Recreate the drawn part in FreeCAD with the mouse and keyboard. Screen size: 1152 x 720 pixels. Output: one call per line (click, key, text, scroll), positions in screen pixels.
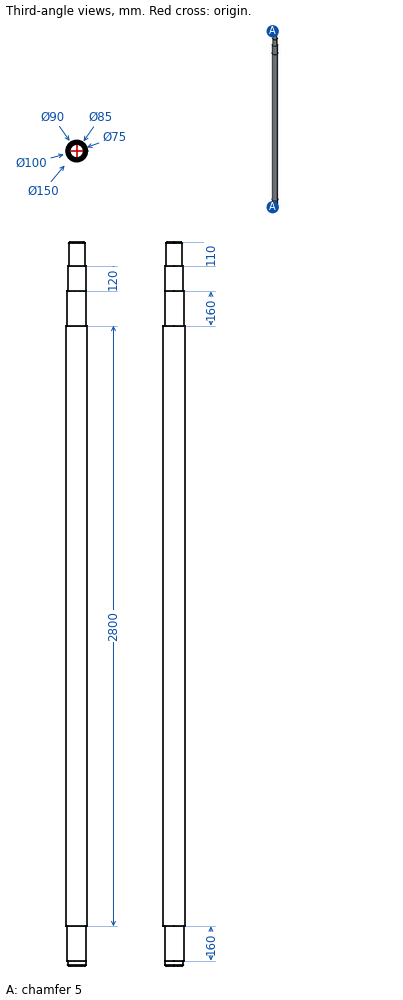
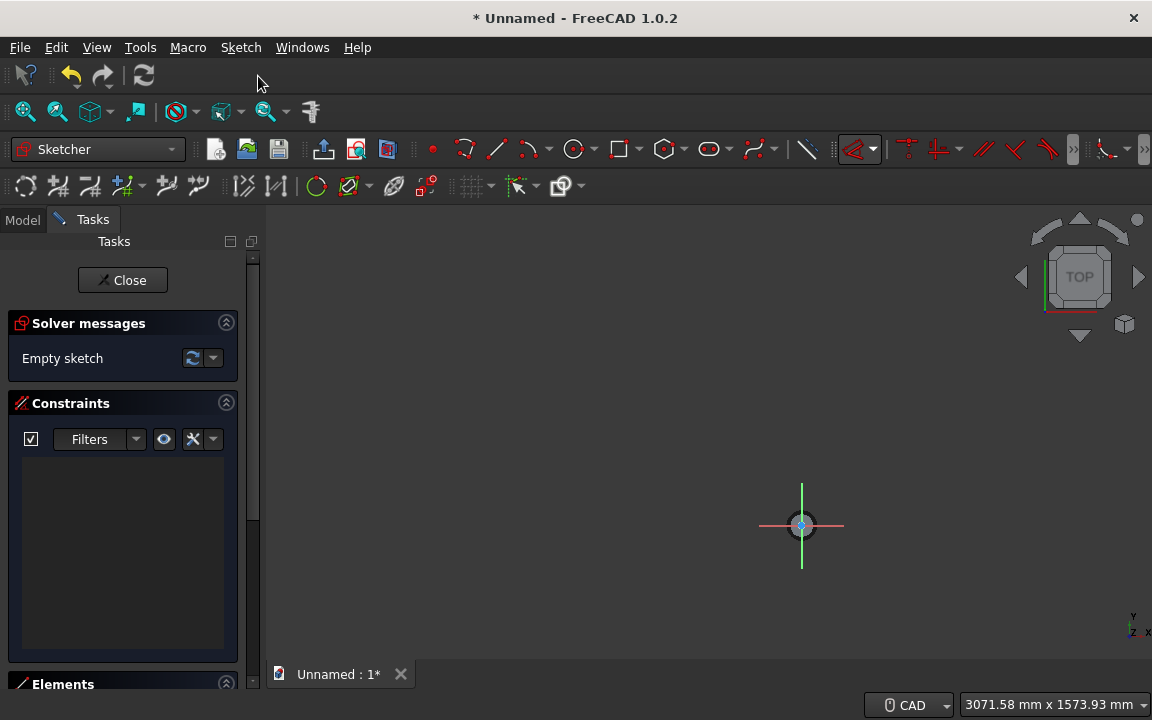
scroll(815, 533, up, 13)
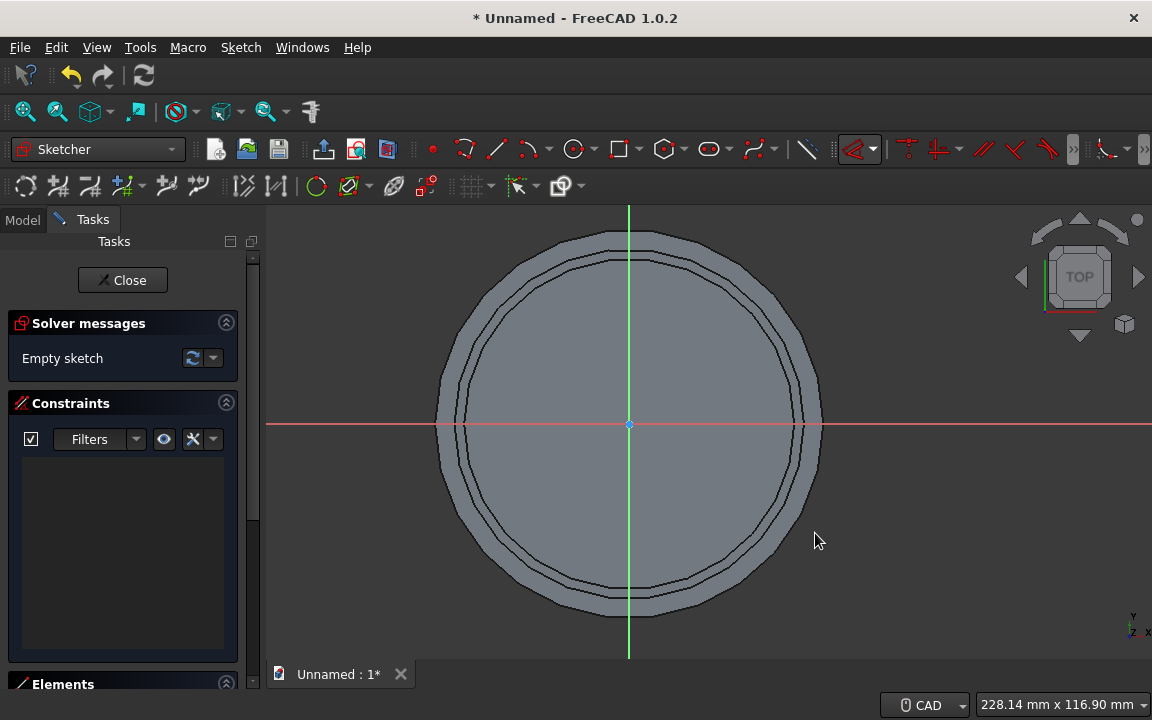
key(g)
key(c)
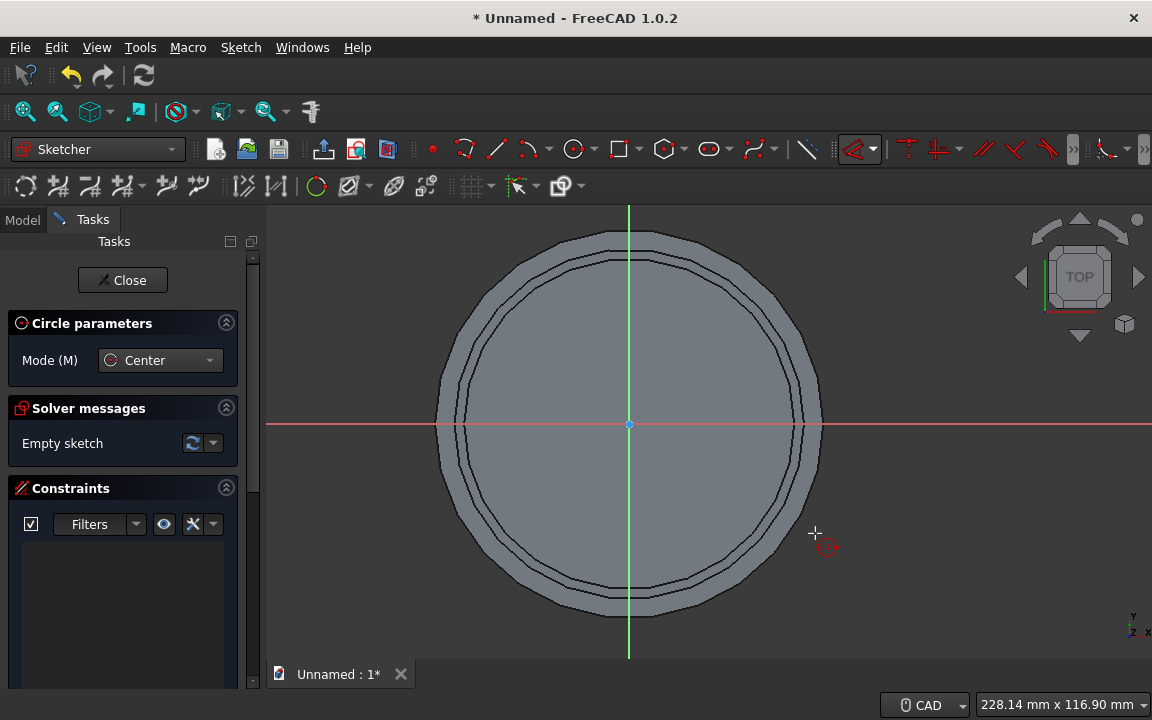
click(629, 424)
click(732, 321)
key(Escape)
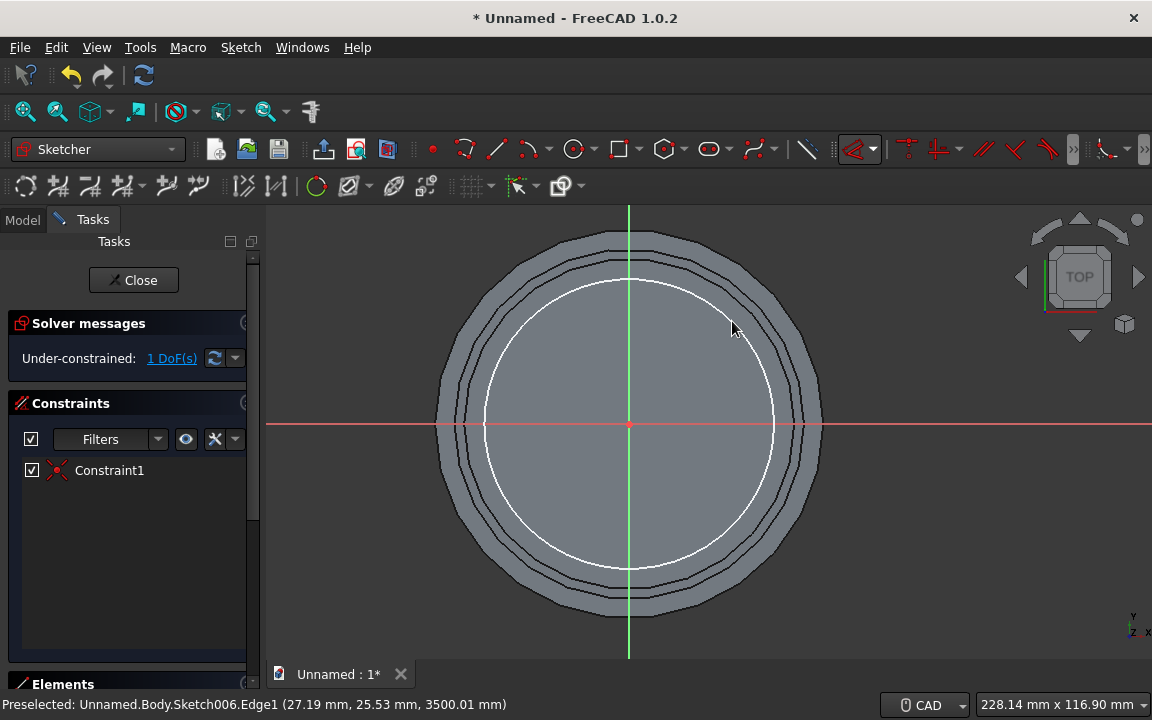
click(731, 321)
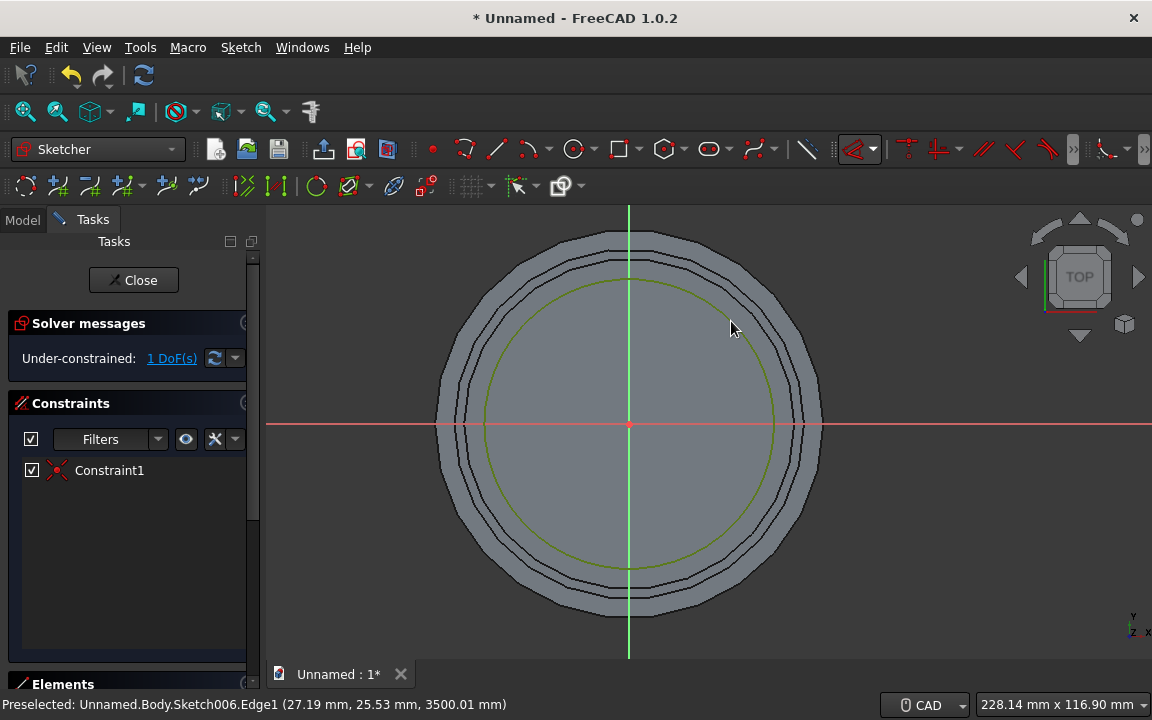
click(876, 150)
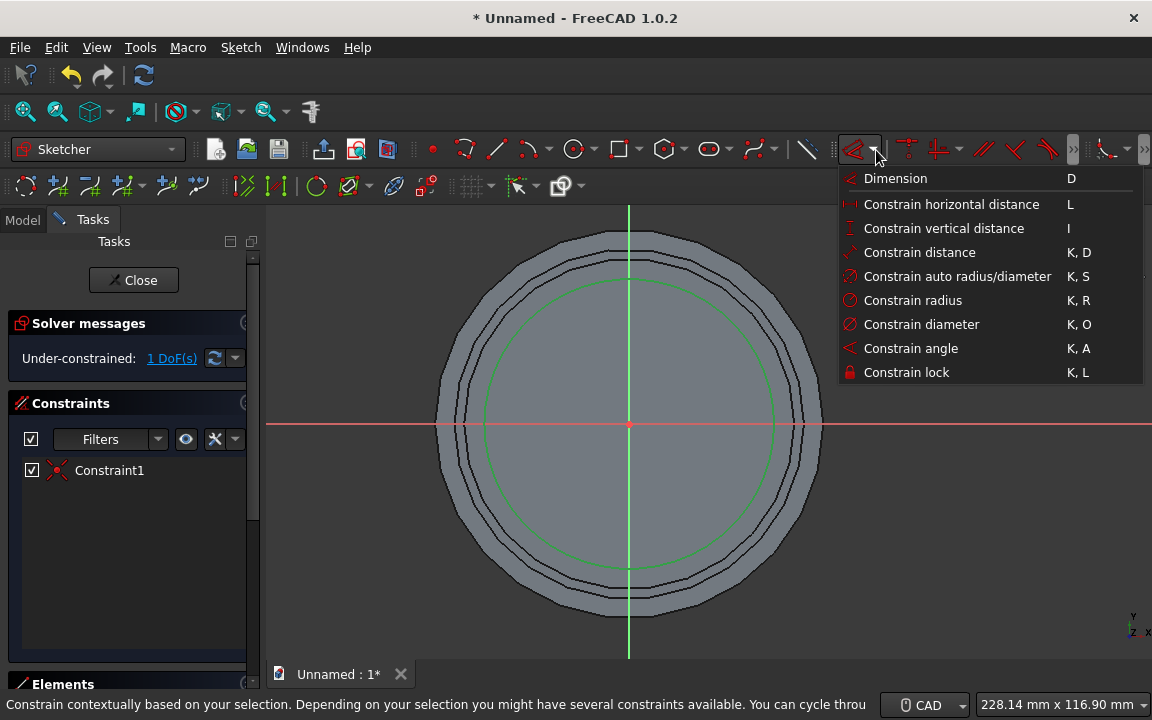
click(991, 324)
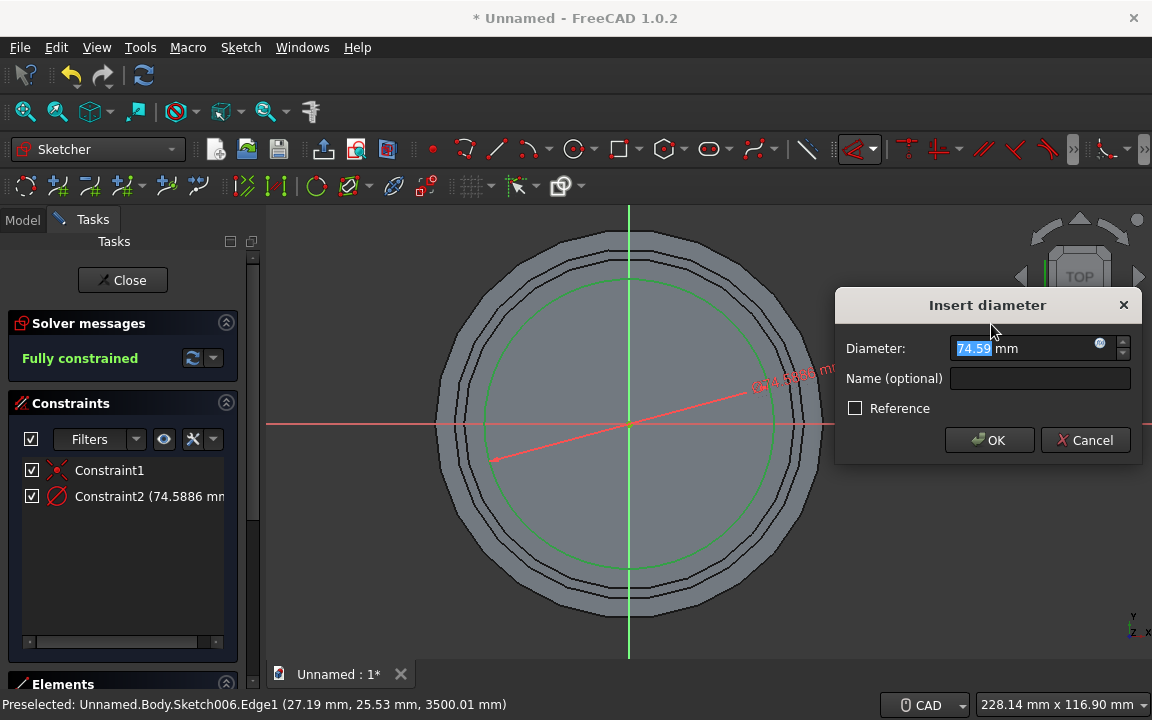
text(75)
key(Return)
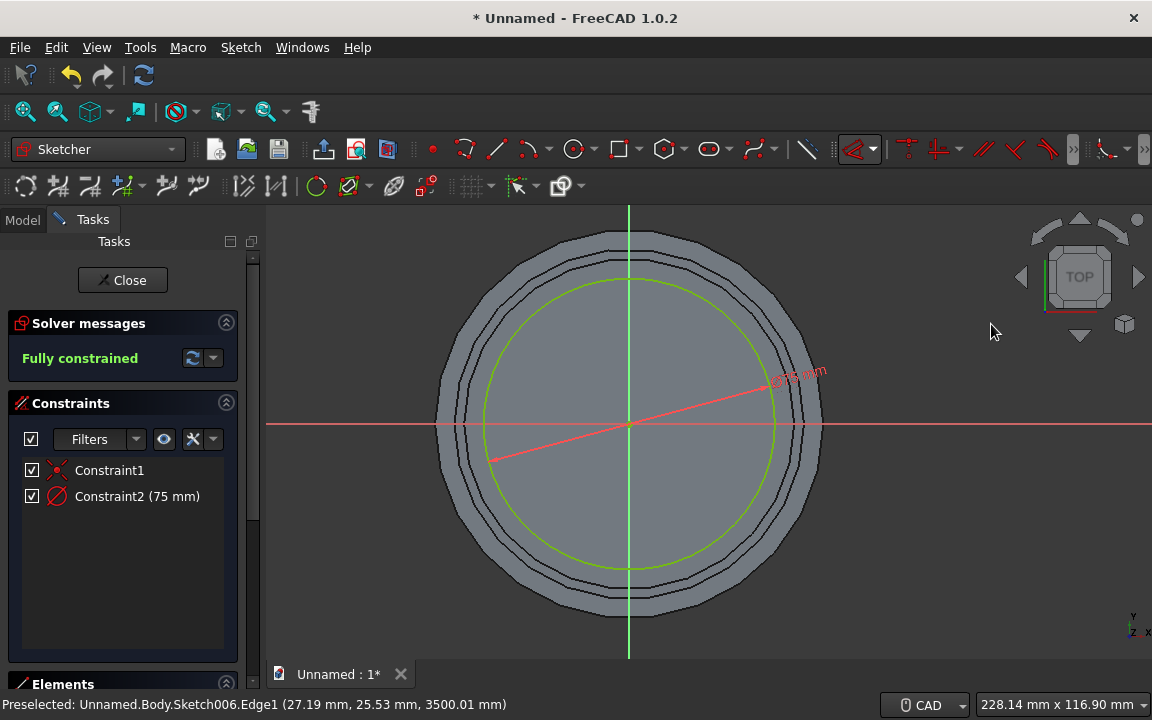
click(123, 280)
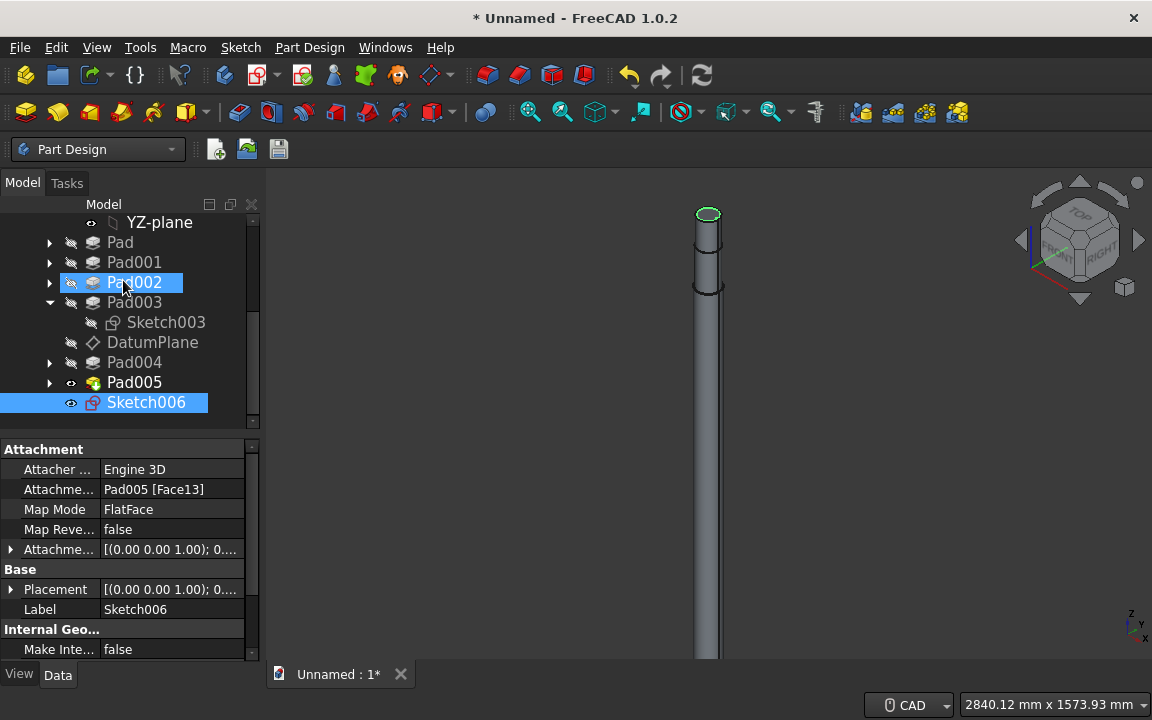
click(26, 112)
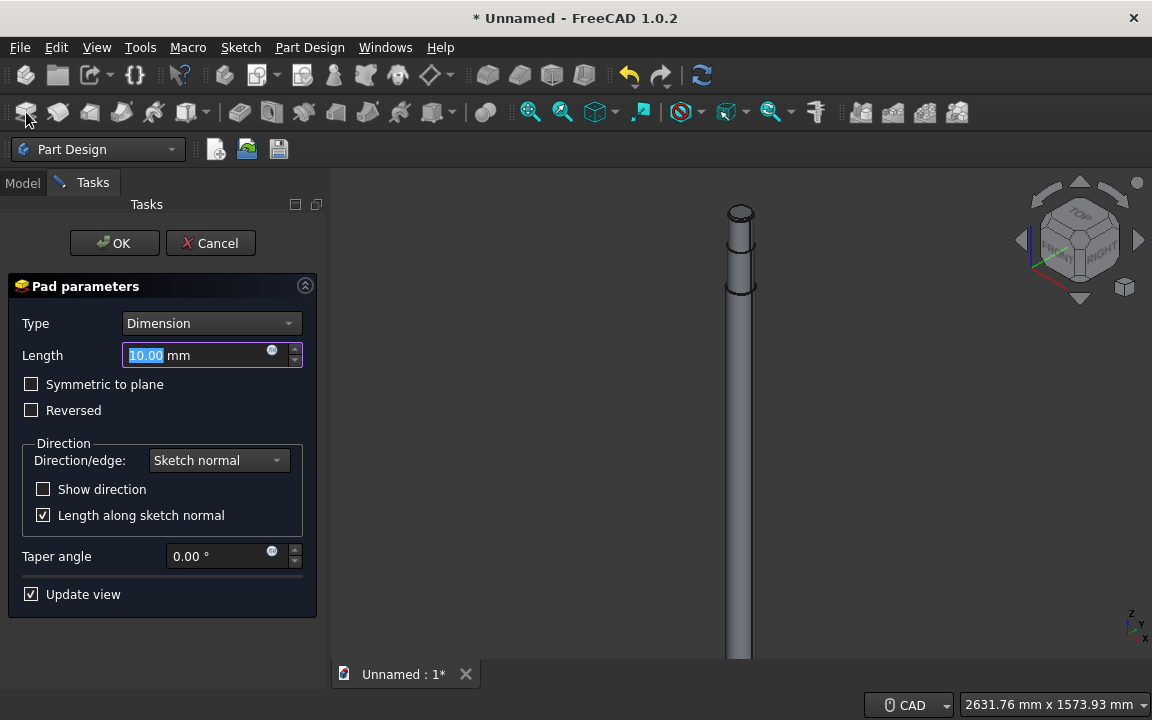
text(110)
key(Tab)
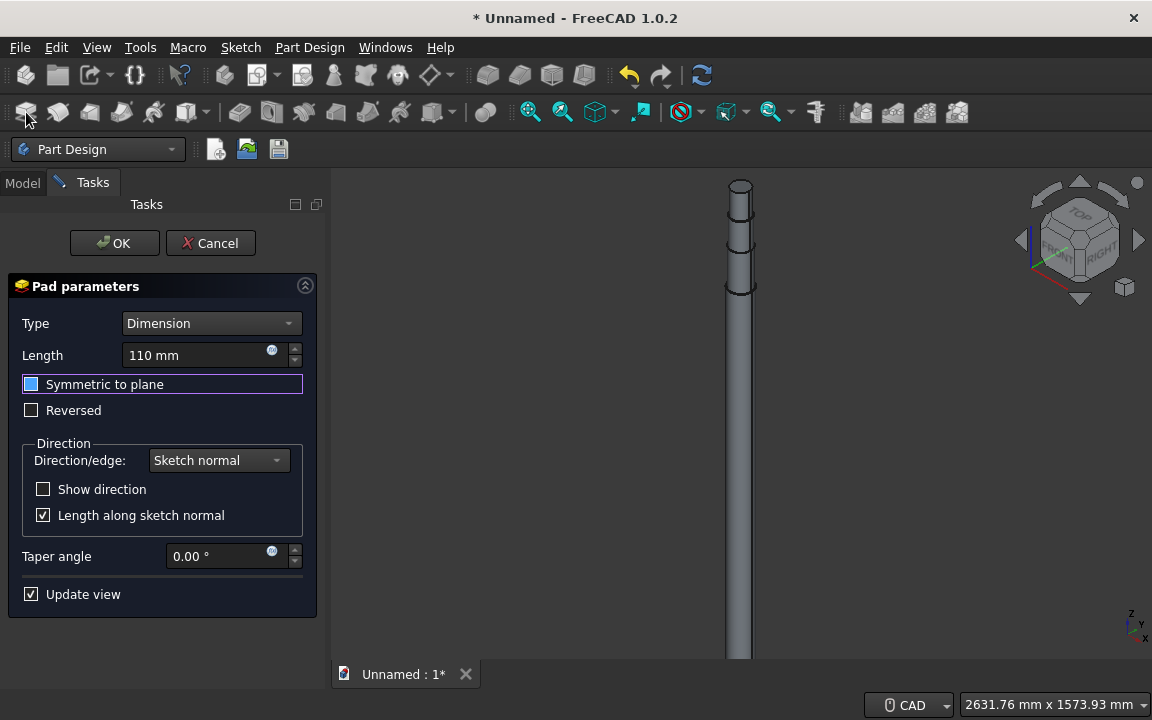
click(115, 243)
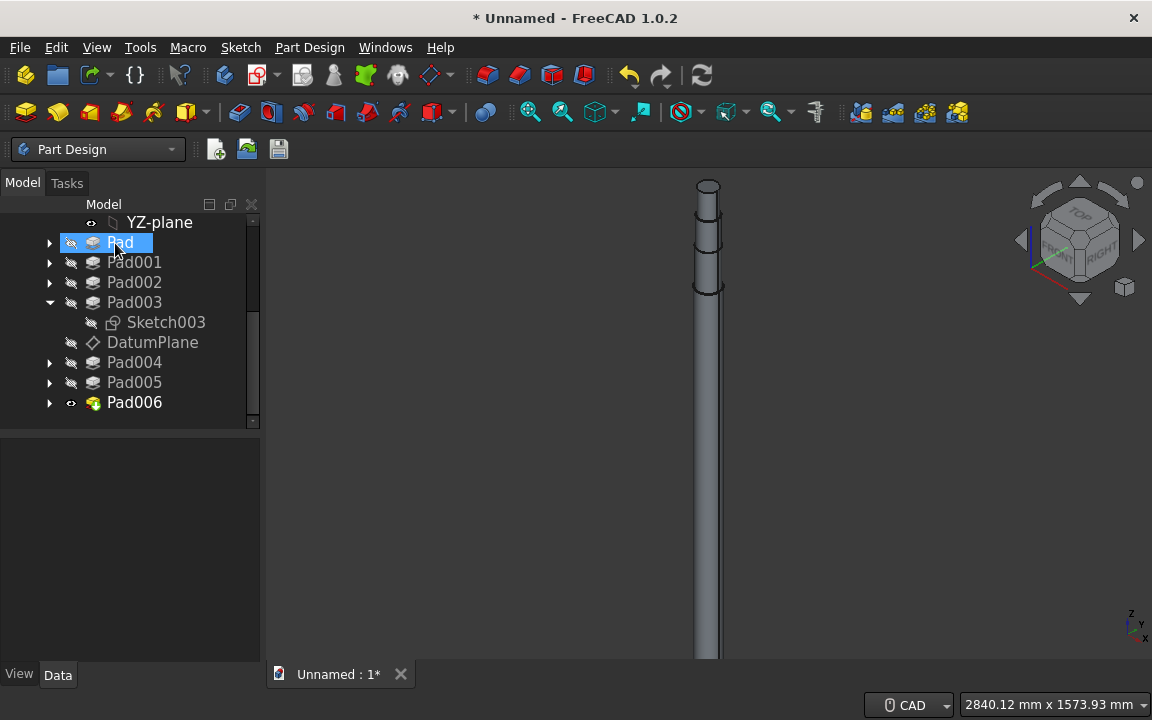
click(532, 112)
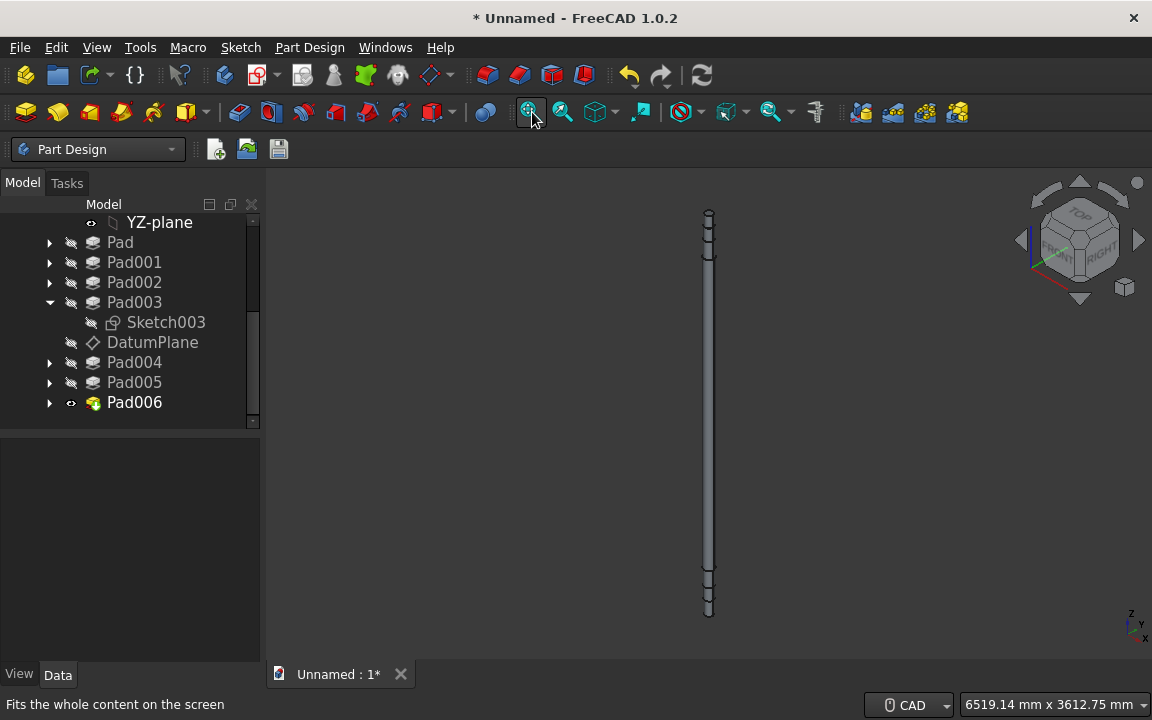
click(258, 76)